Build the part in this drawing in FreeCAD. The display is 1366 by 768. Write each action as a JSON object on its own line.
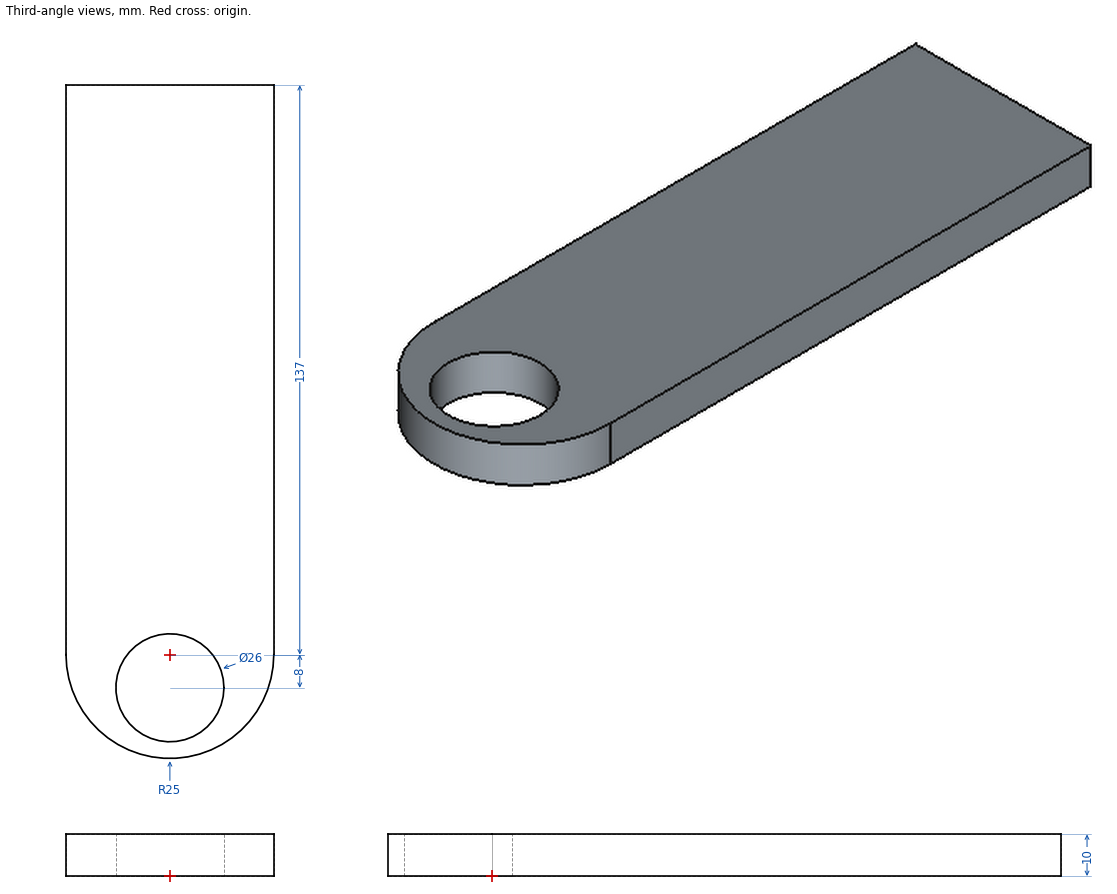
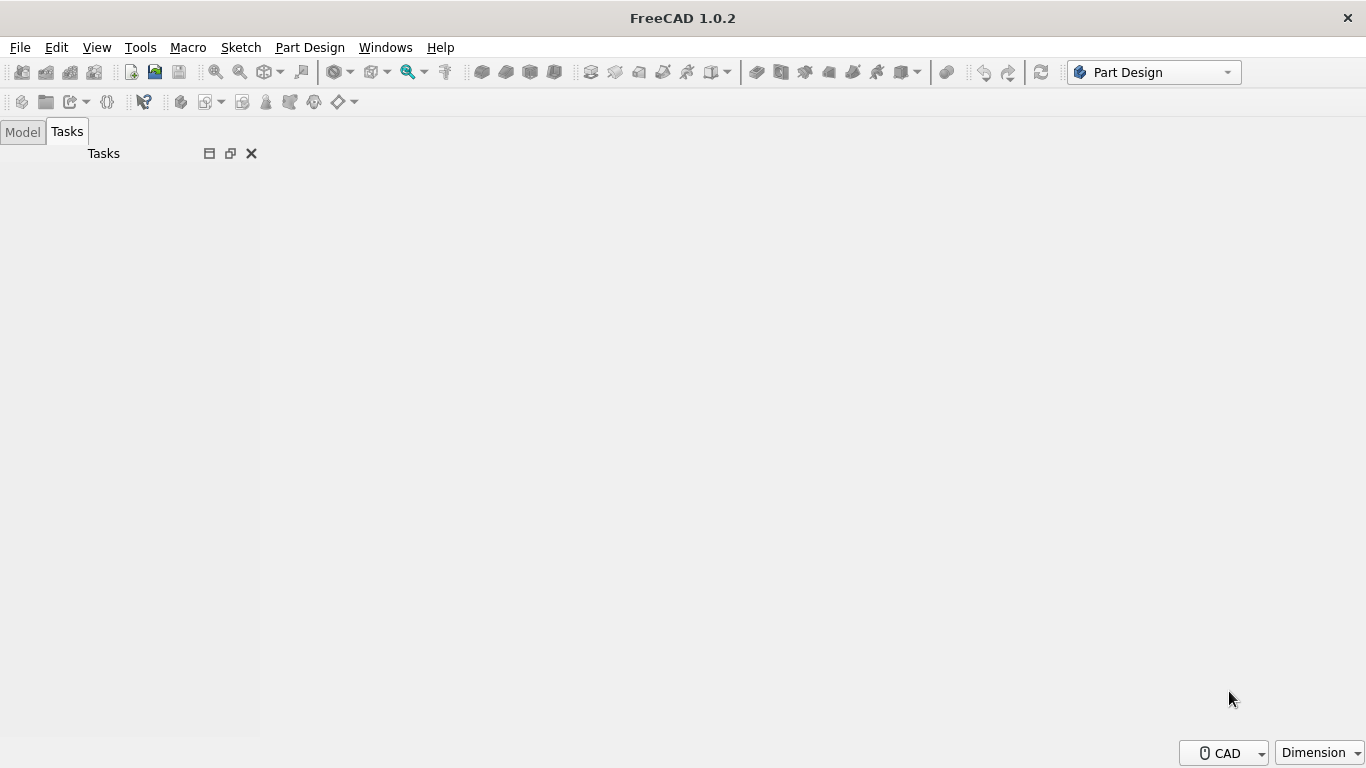
{"action": "left_click", "coordinate": [132, 72]}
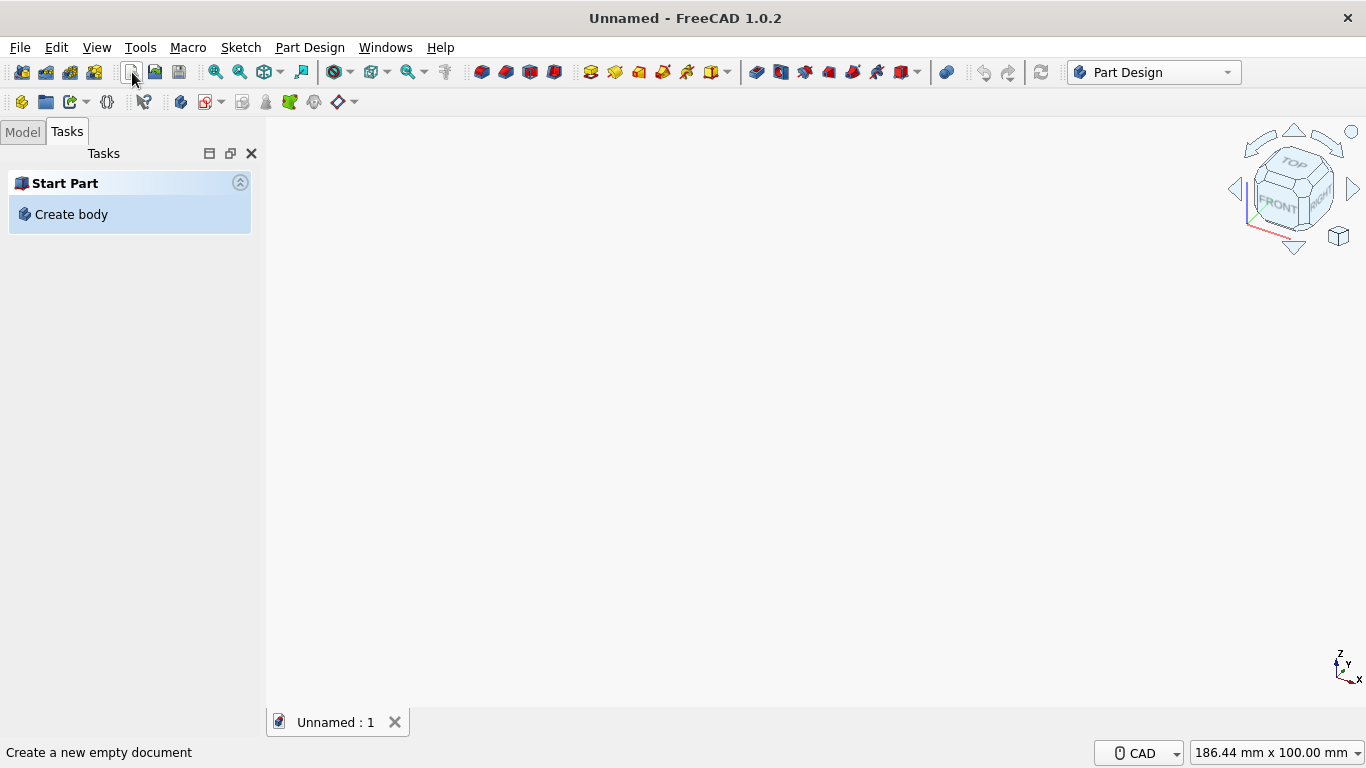
{"action": "left_click", "coordinate": [206, 102]}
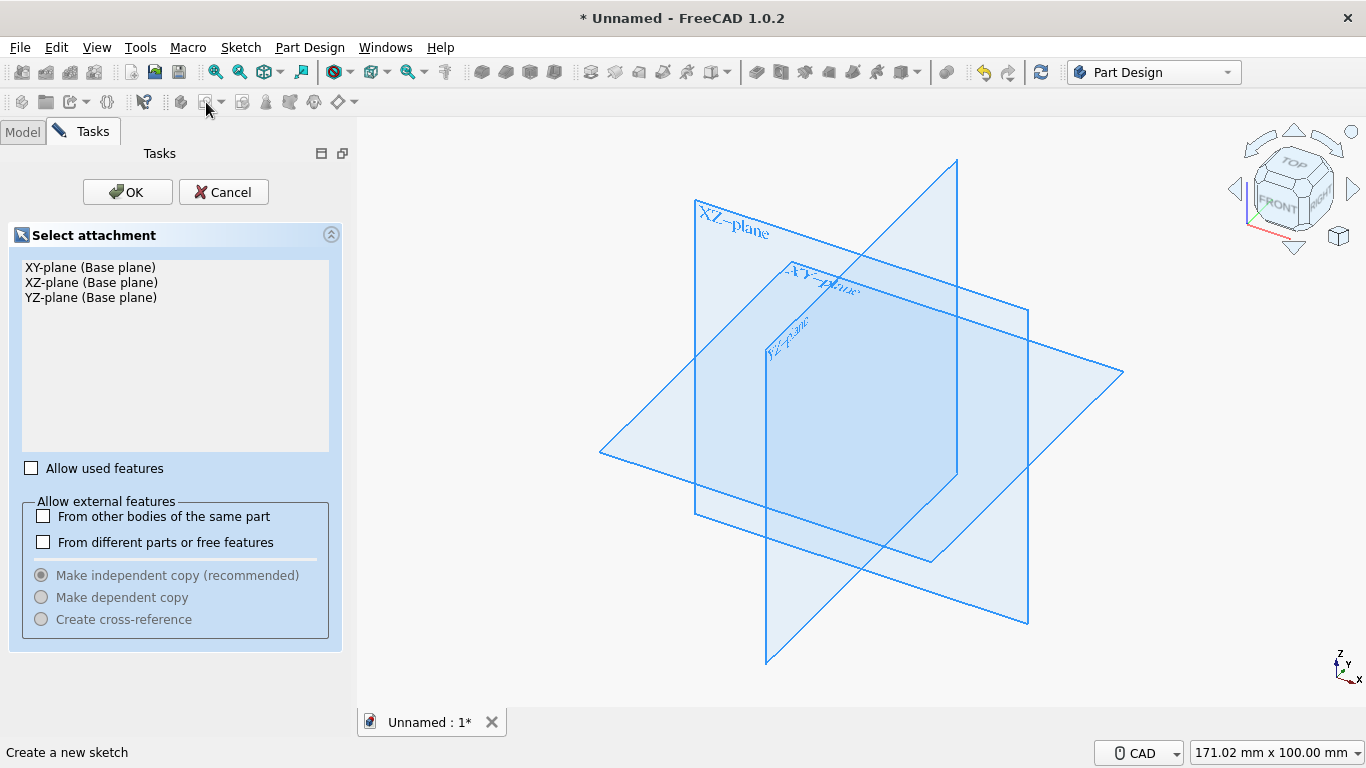
{"action": "left_click", "coordinate": [82, 268]}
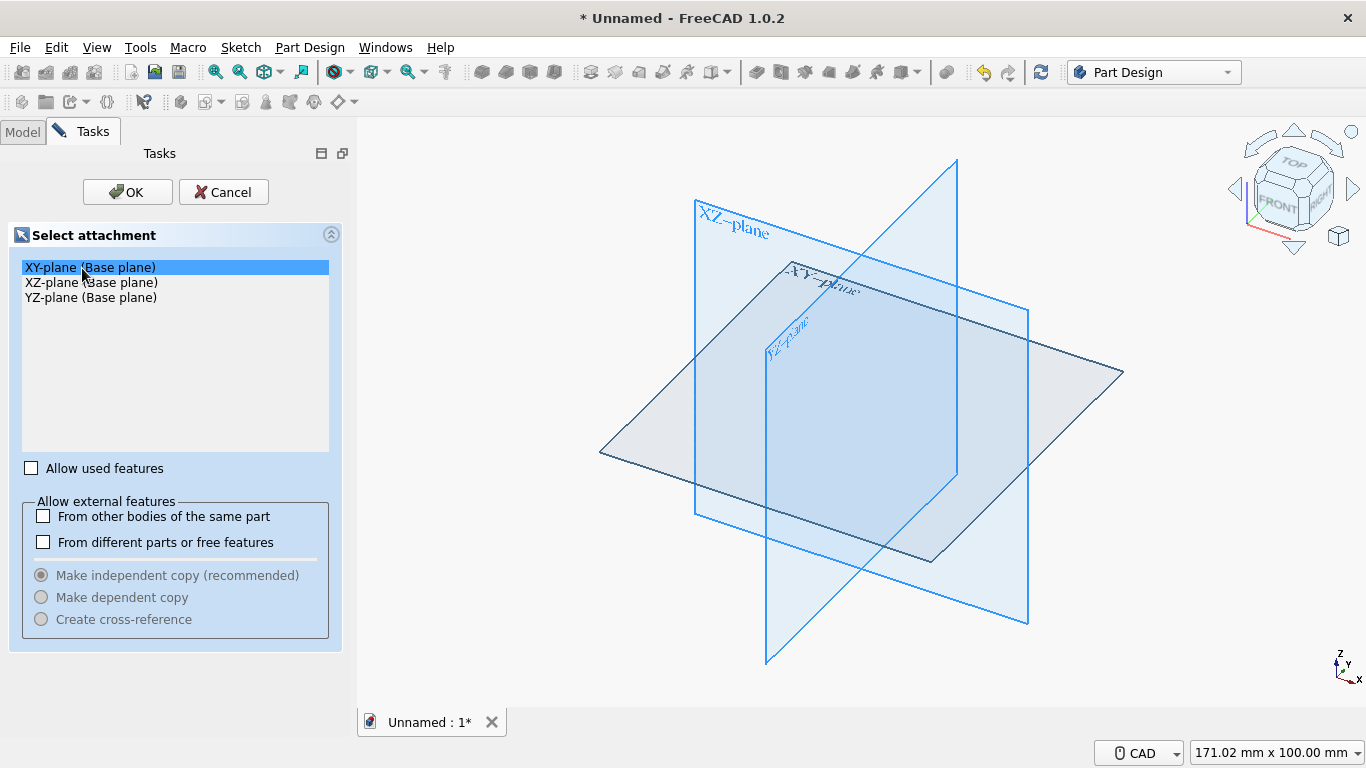
{"action": "left_click", "coordinate": [128, 192]}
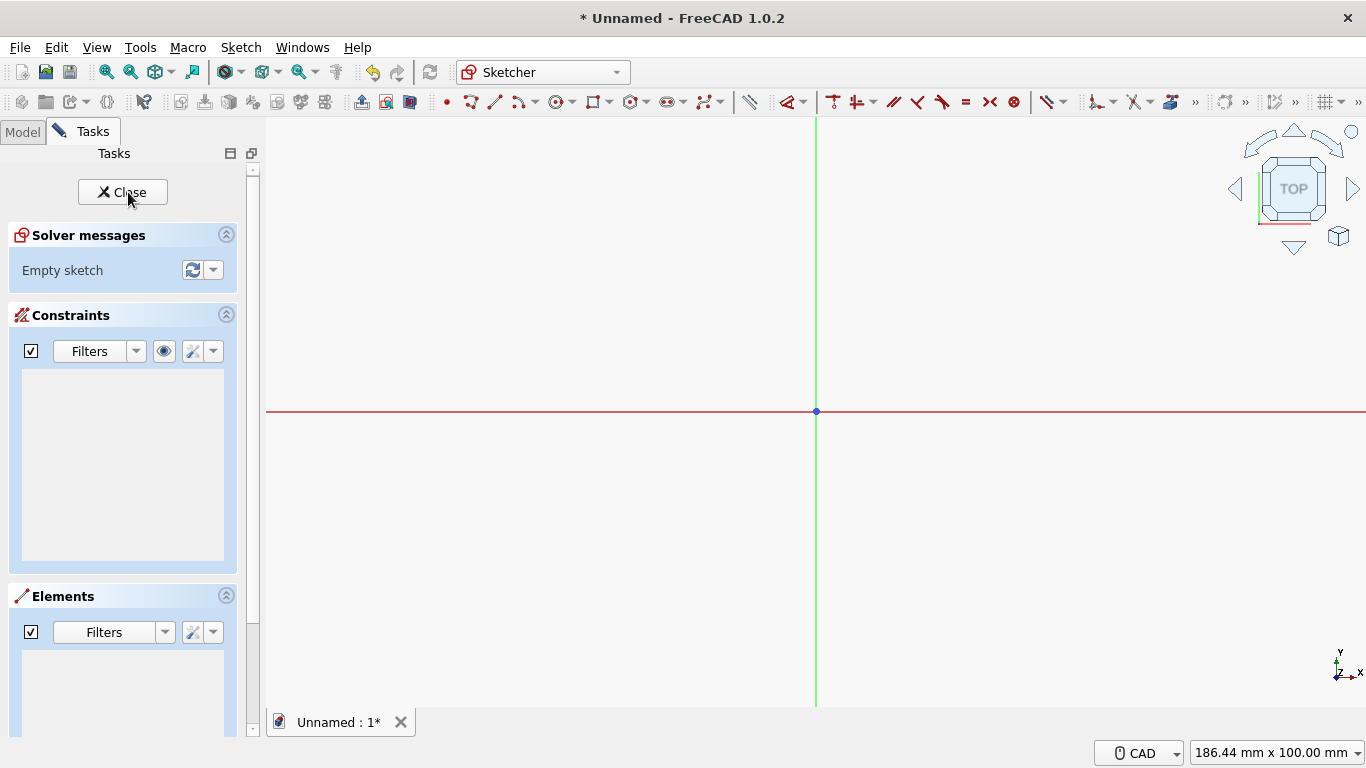
{"action": "scroll", "coordinate": [708, 604], "scroll_direction": "down", "scroll_amount": 5}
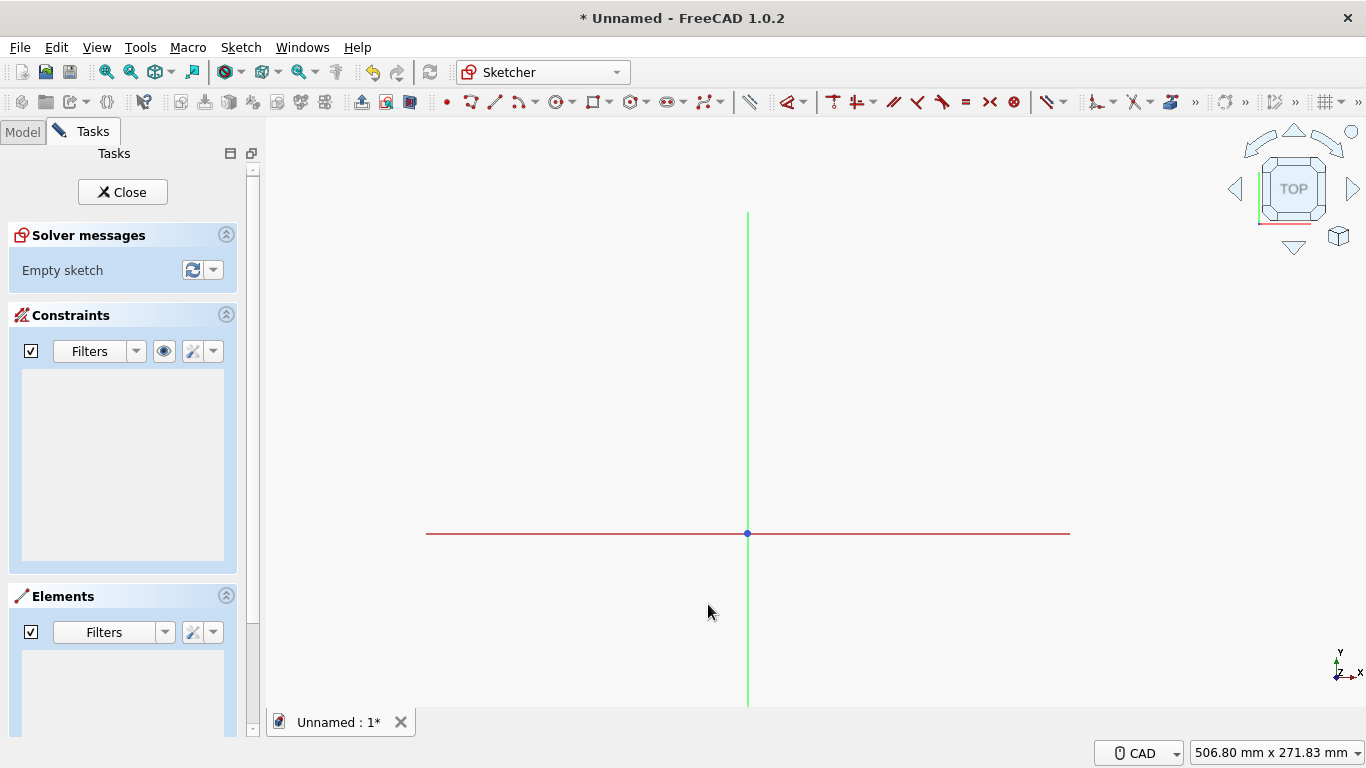
{"action": "left_click", "coordinate": [472, 102]}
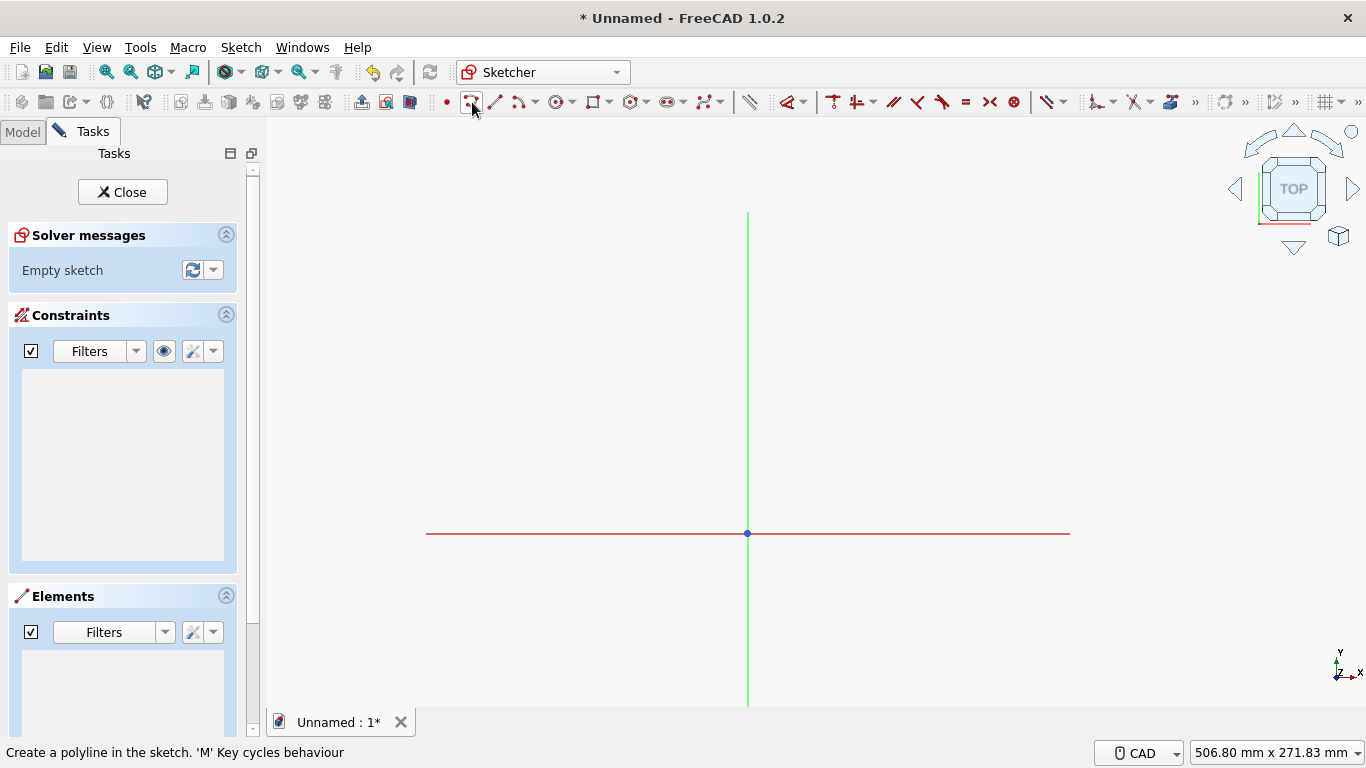
{"action": "left_click", "coordinate": [802, 534]}
{"action": "left_click", "coordinate": [802, 237]}
{"action": "left_click", "coordinate": [694, 237]}
{"action": "left_click", "coordinate": [694, 534]}
{"action": "right_click", "coordinate": [694, 534]}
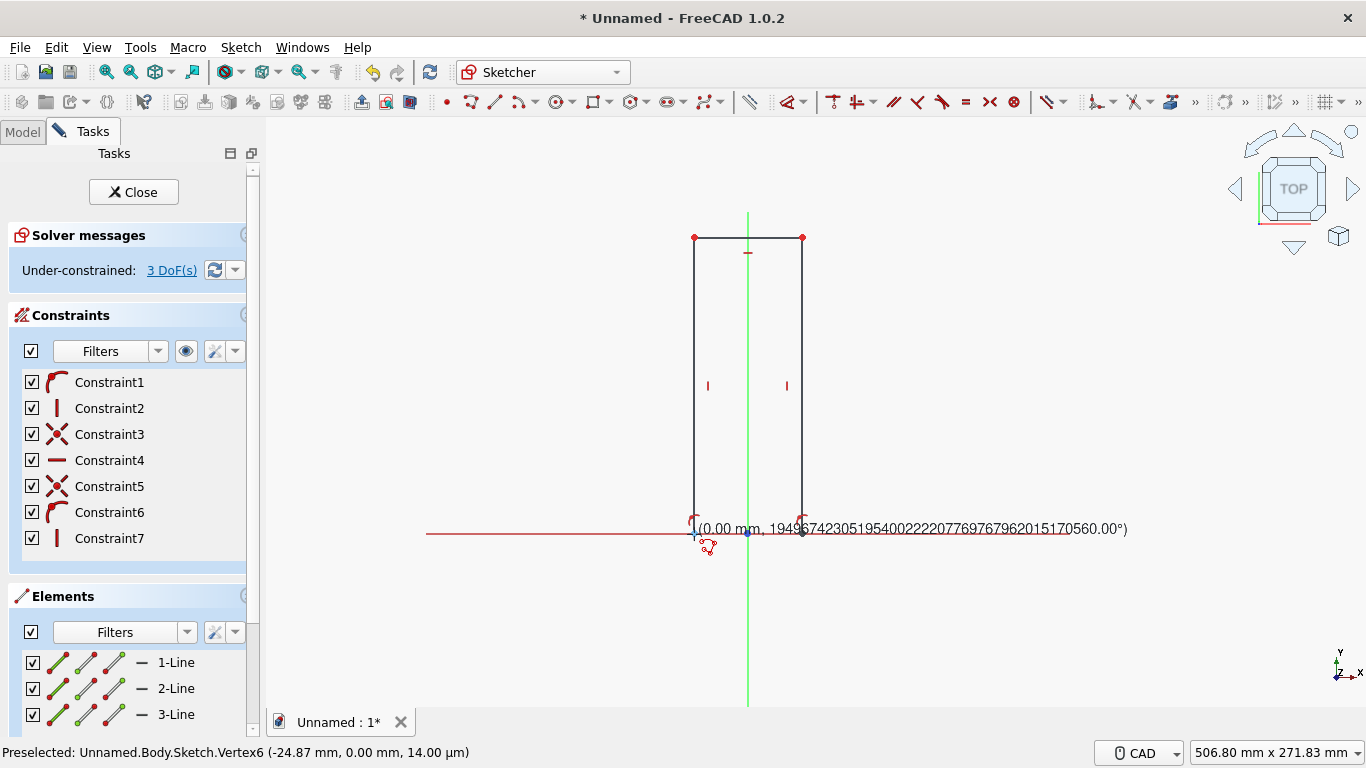
{"action": "key", "text": "g 3 a"}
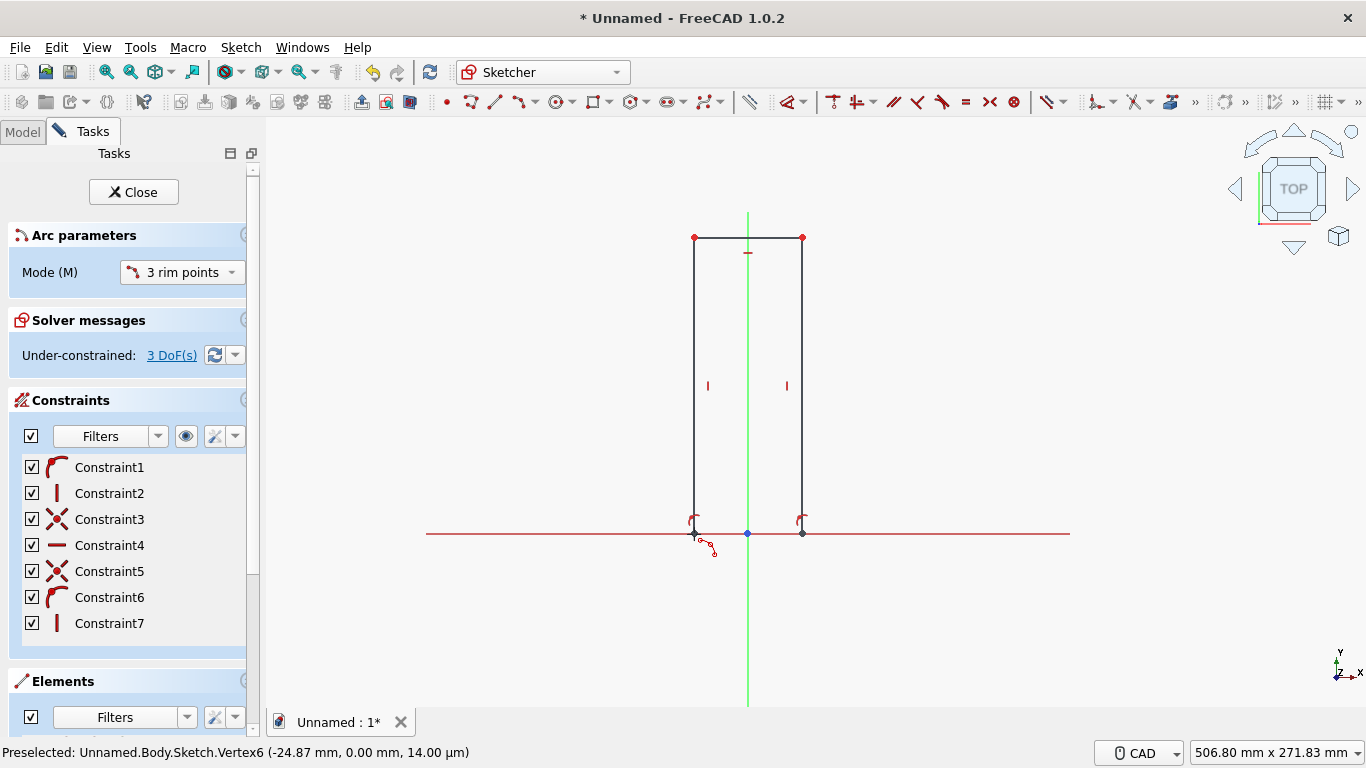
{"action": "left_click", "coordinate": [694, 534]}
{"action": "left_click", "coordinate": [802, 534]}
{"action": "left_click", "coordinate": [731, 585]}
{"action": "key", "text": "Escape"}